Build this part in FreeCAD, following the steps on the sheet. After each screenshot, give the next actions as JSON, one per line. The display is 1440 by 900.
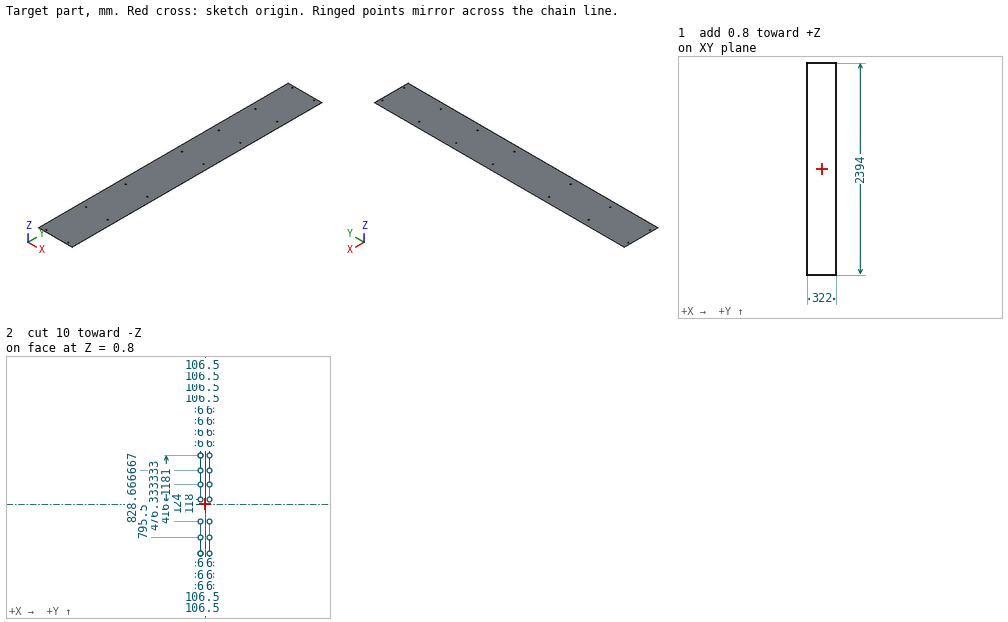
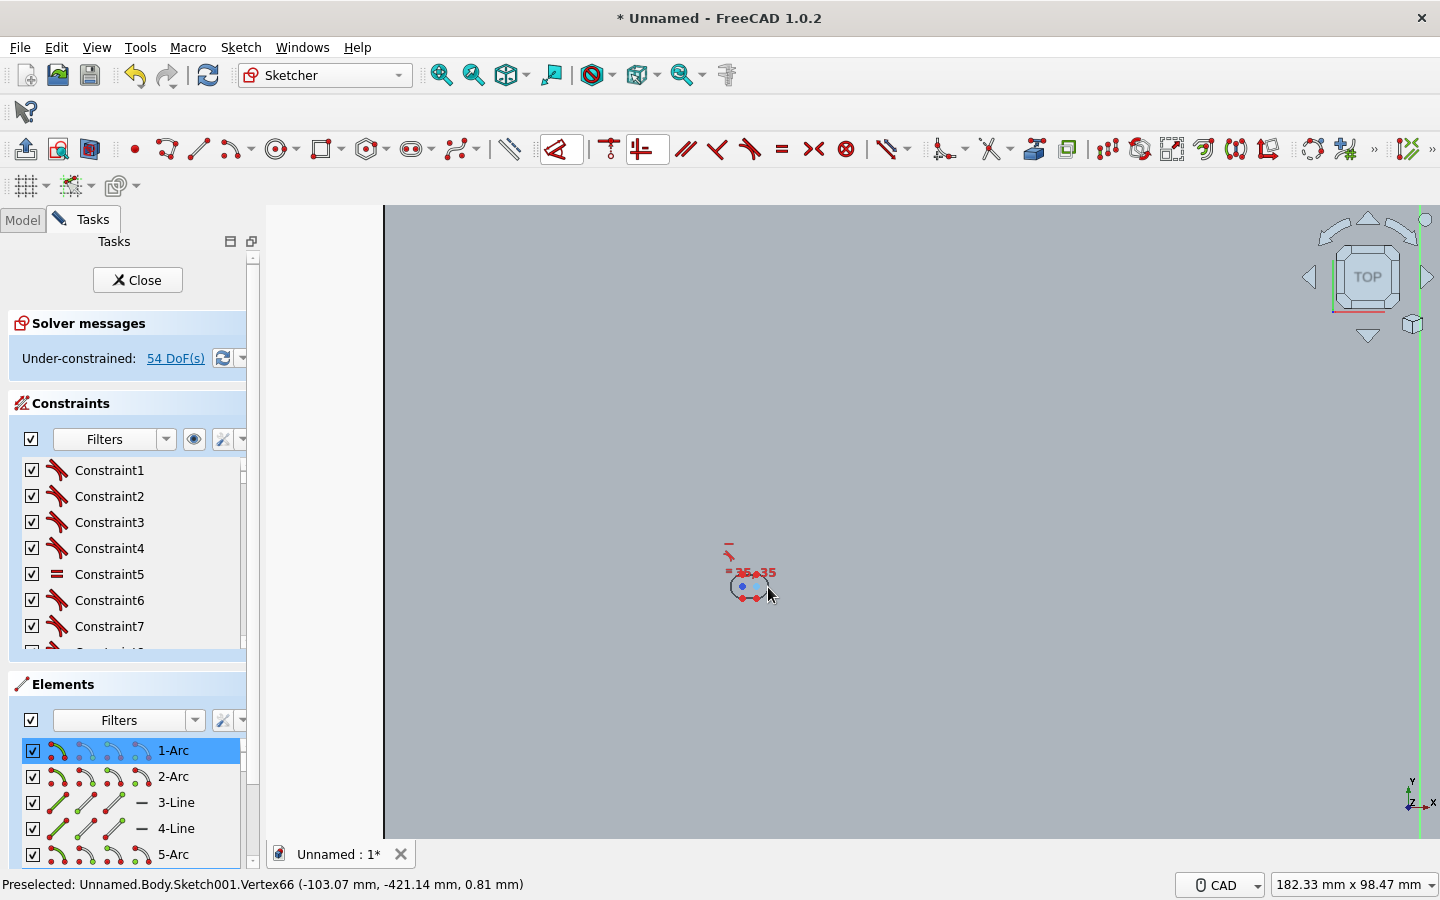
{"action": "left_click", "coordinate": [768, 586]}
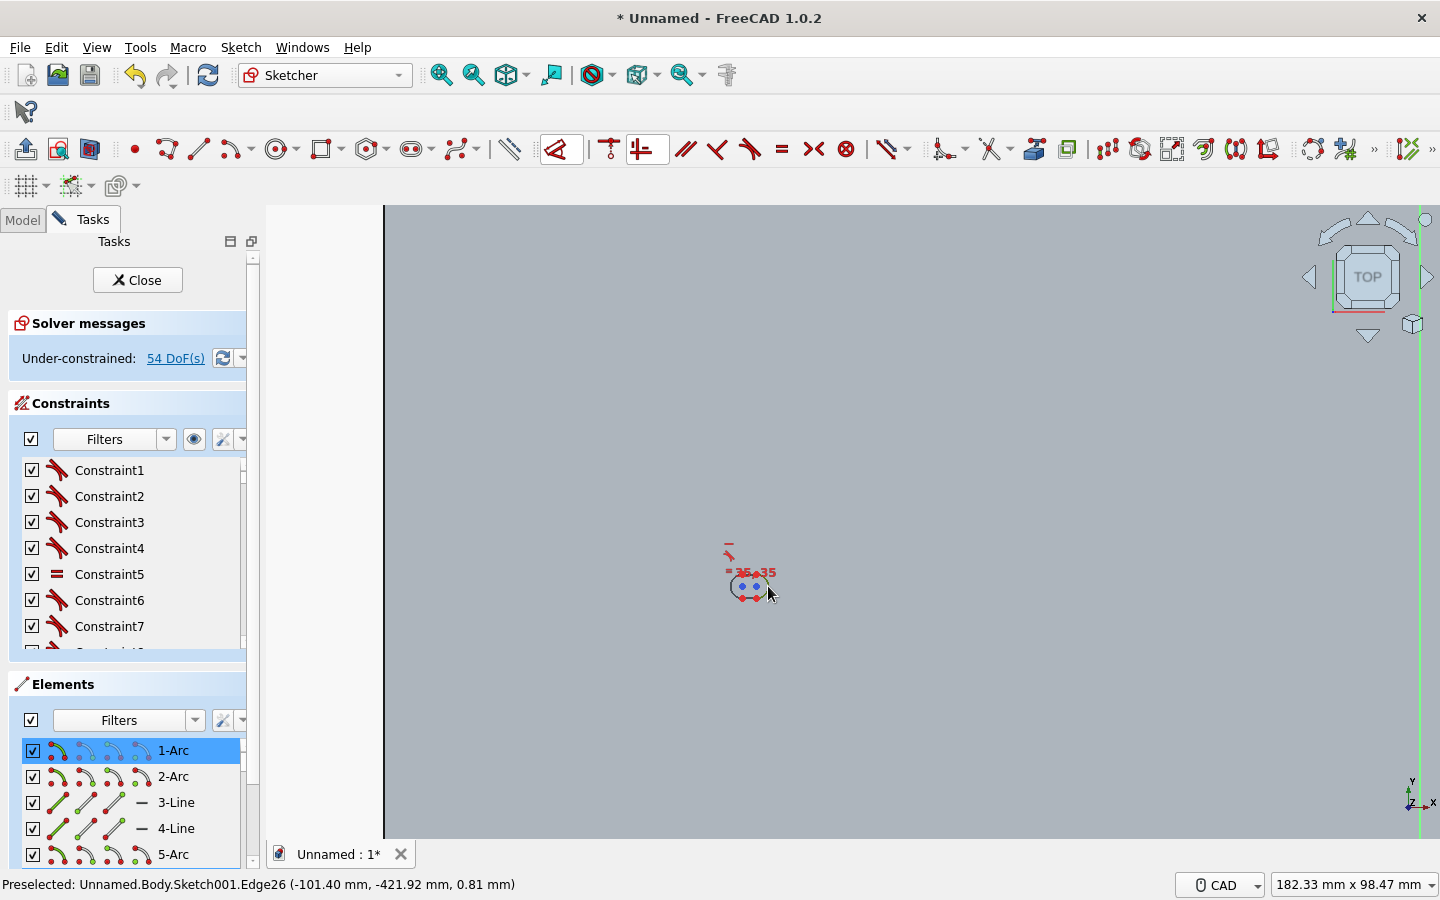
{"action": "scroll", "coordinate": [763, 613], "scroll_direction": "down", "scroll_amount": 17}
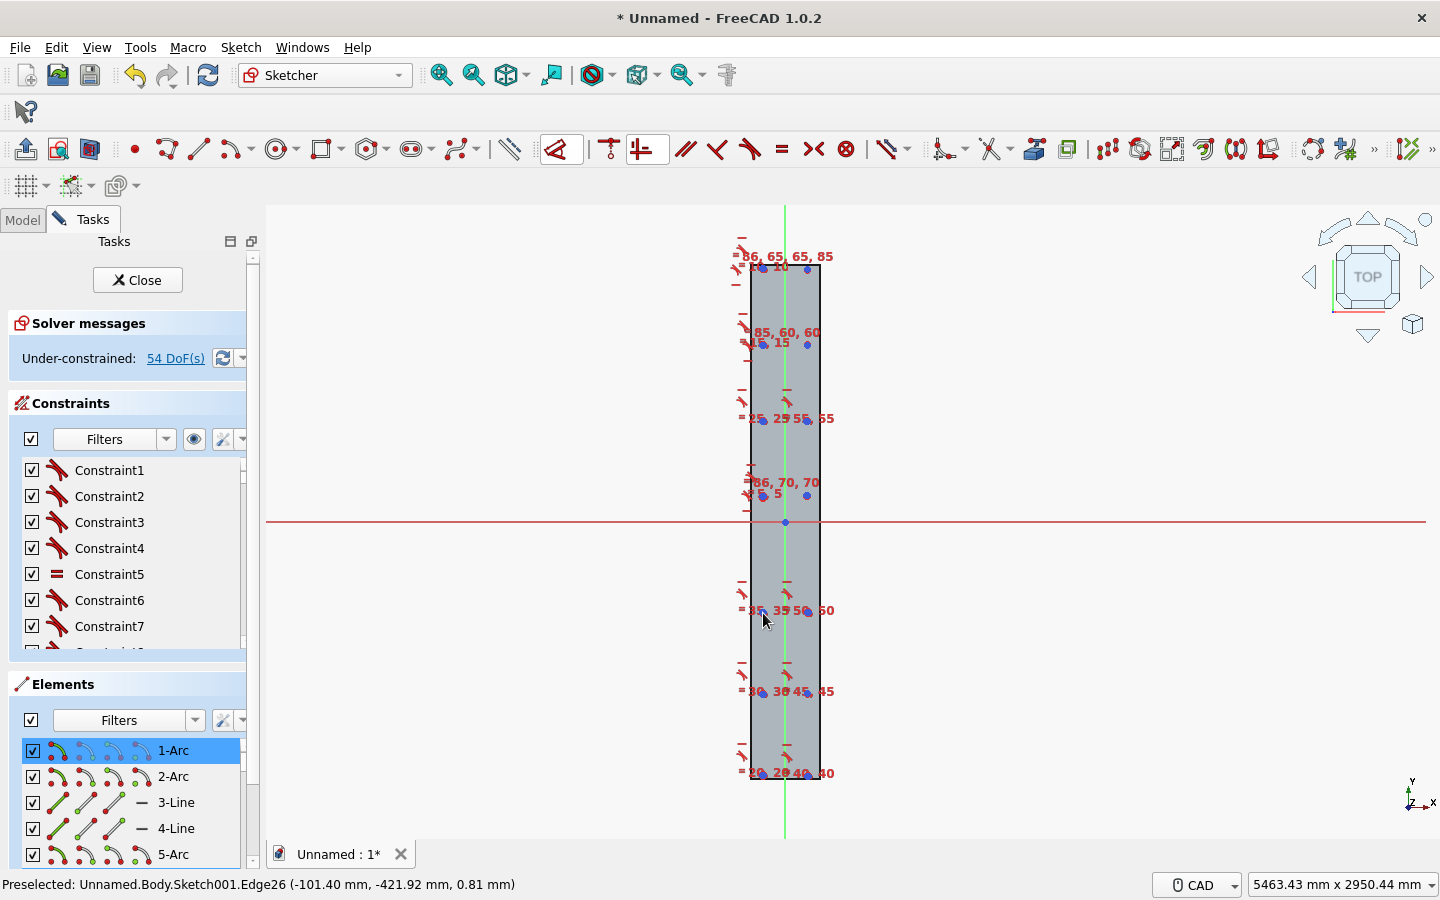
{"action": "scroll", "coordinate": [809, 777], "scroll_direction": "up", "scroll_amount": 13}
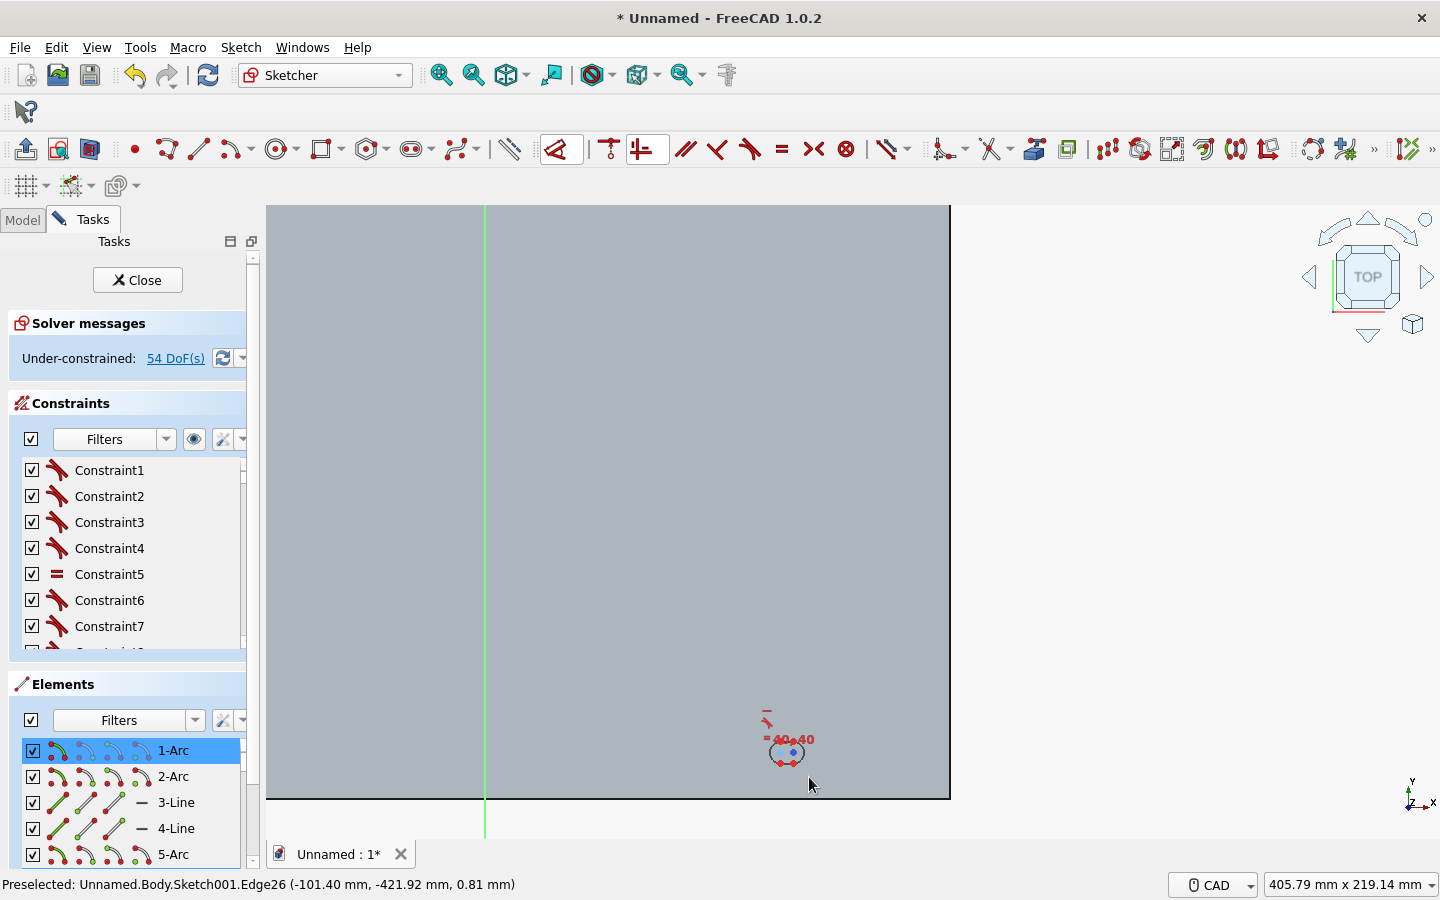
{"action": "left_click", "coordinate": [802, 759]}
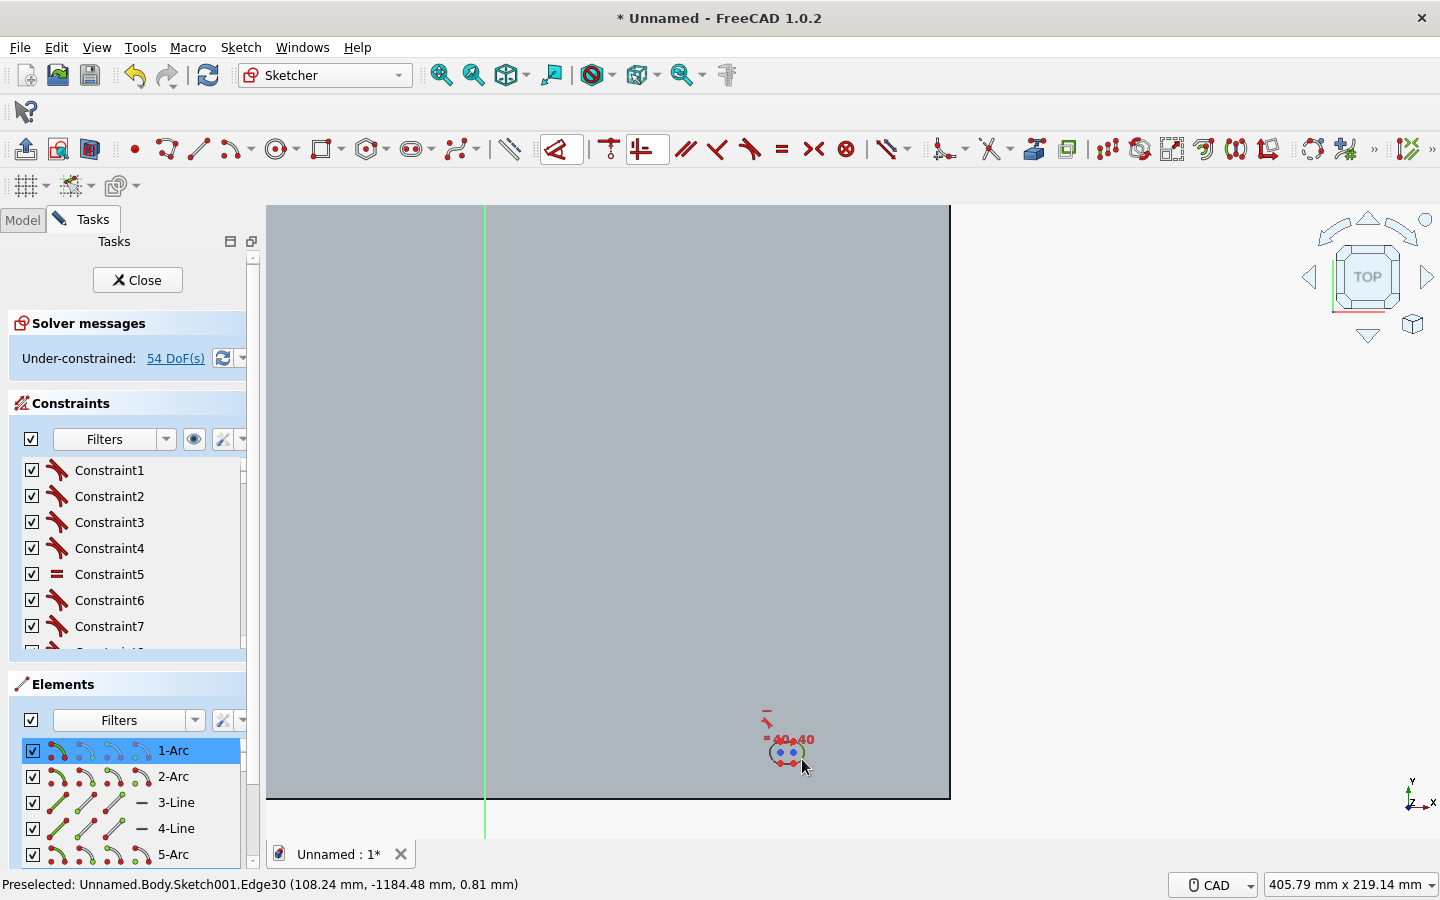
{"action": "scroll", "coordinate": [804, 728], "scroll_direction": "down", "scroll_amount": 14}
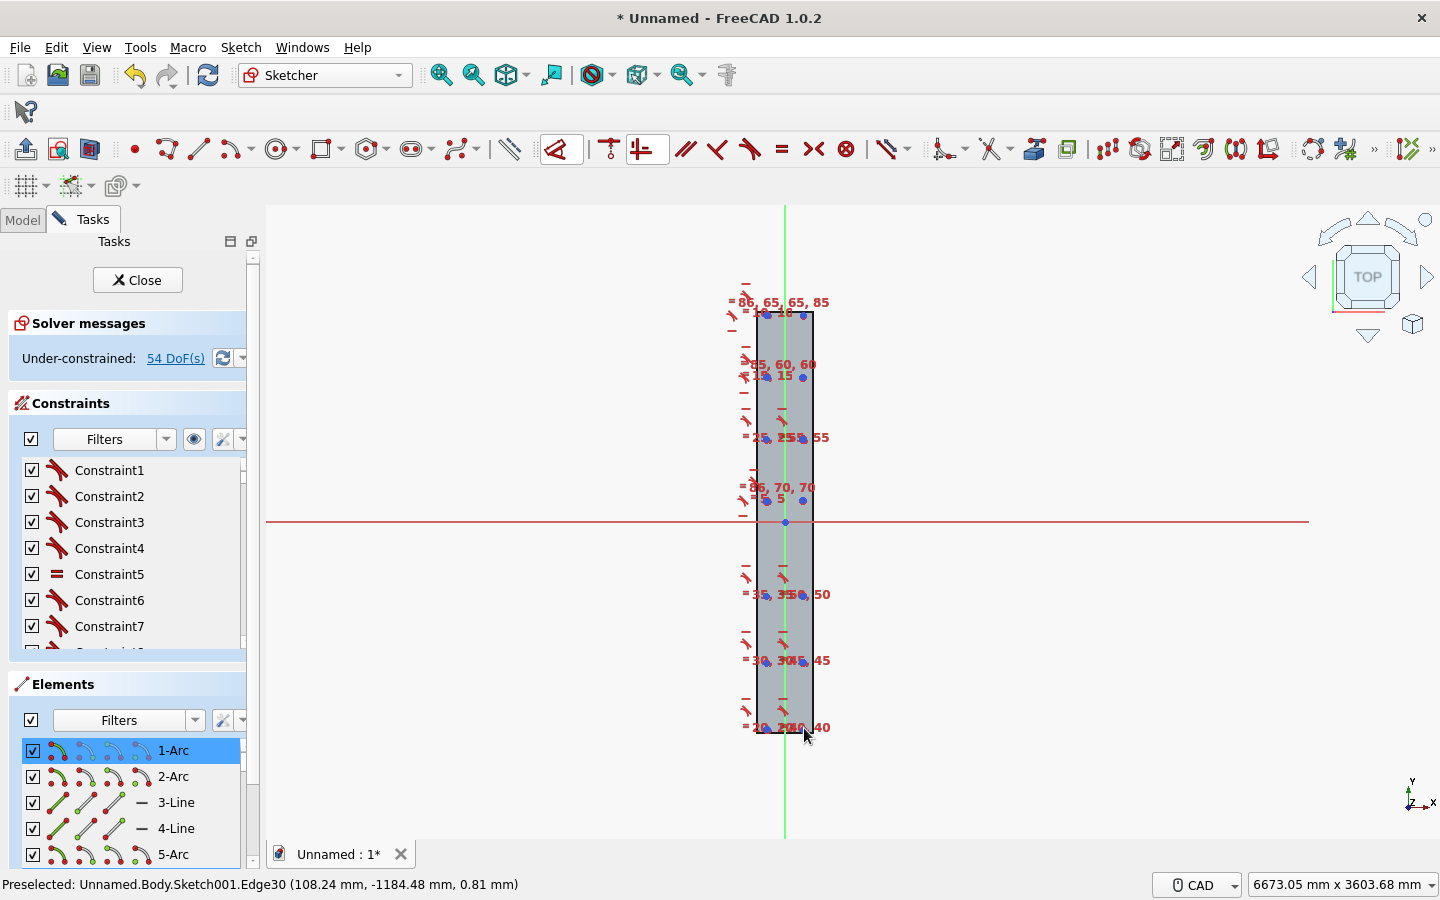
{"action": "scroll", "coordinate": [804, 663], "scroll_direction": "up", "scroll_amount": 14}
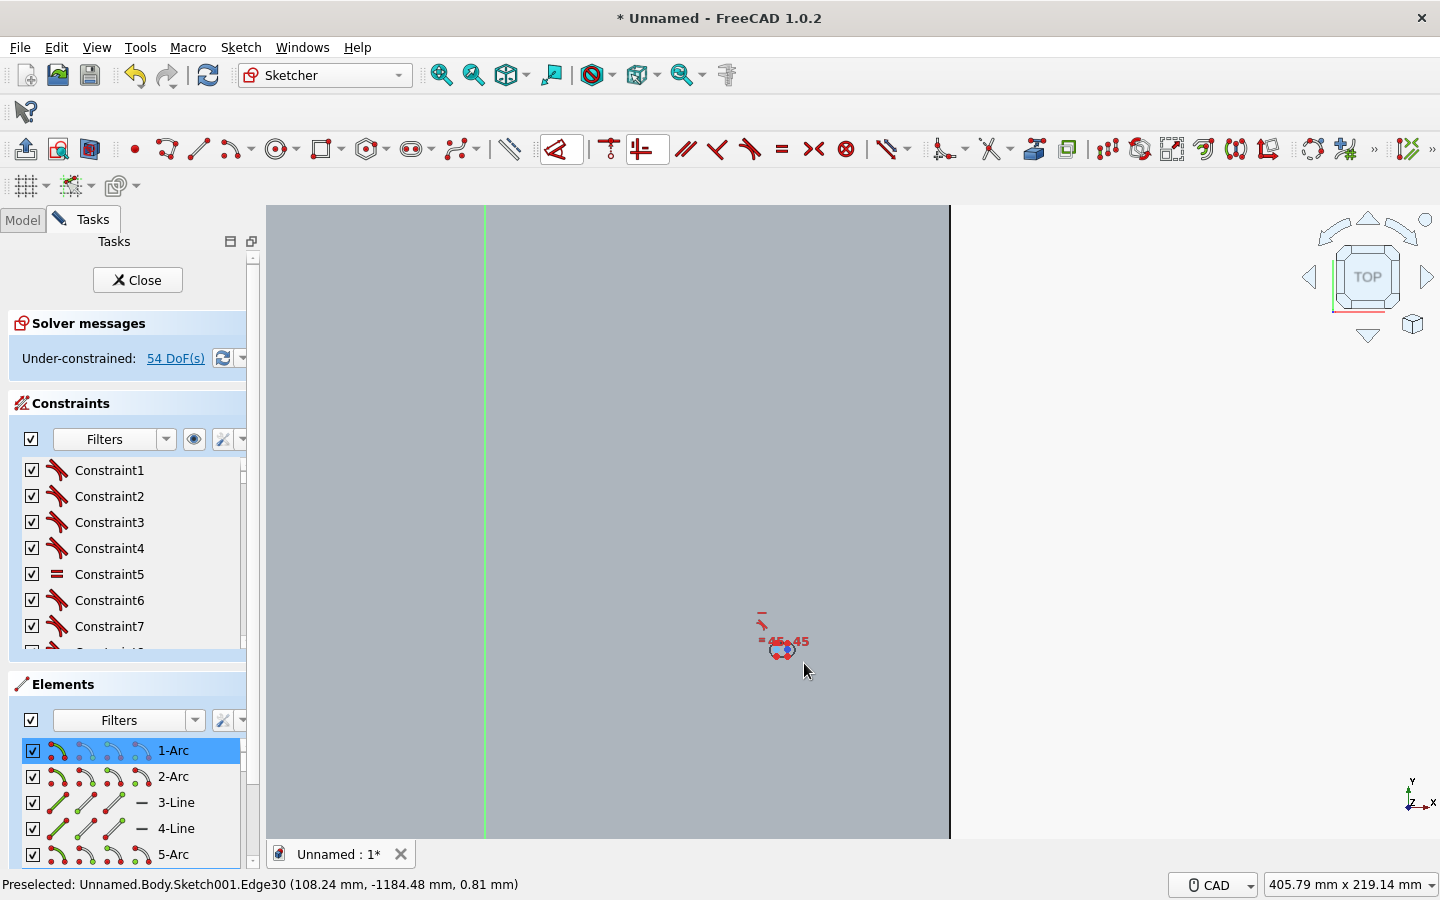
{"action": "left_click", "coordinate": [795, 650]}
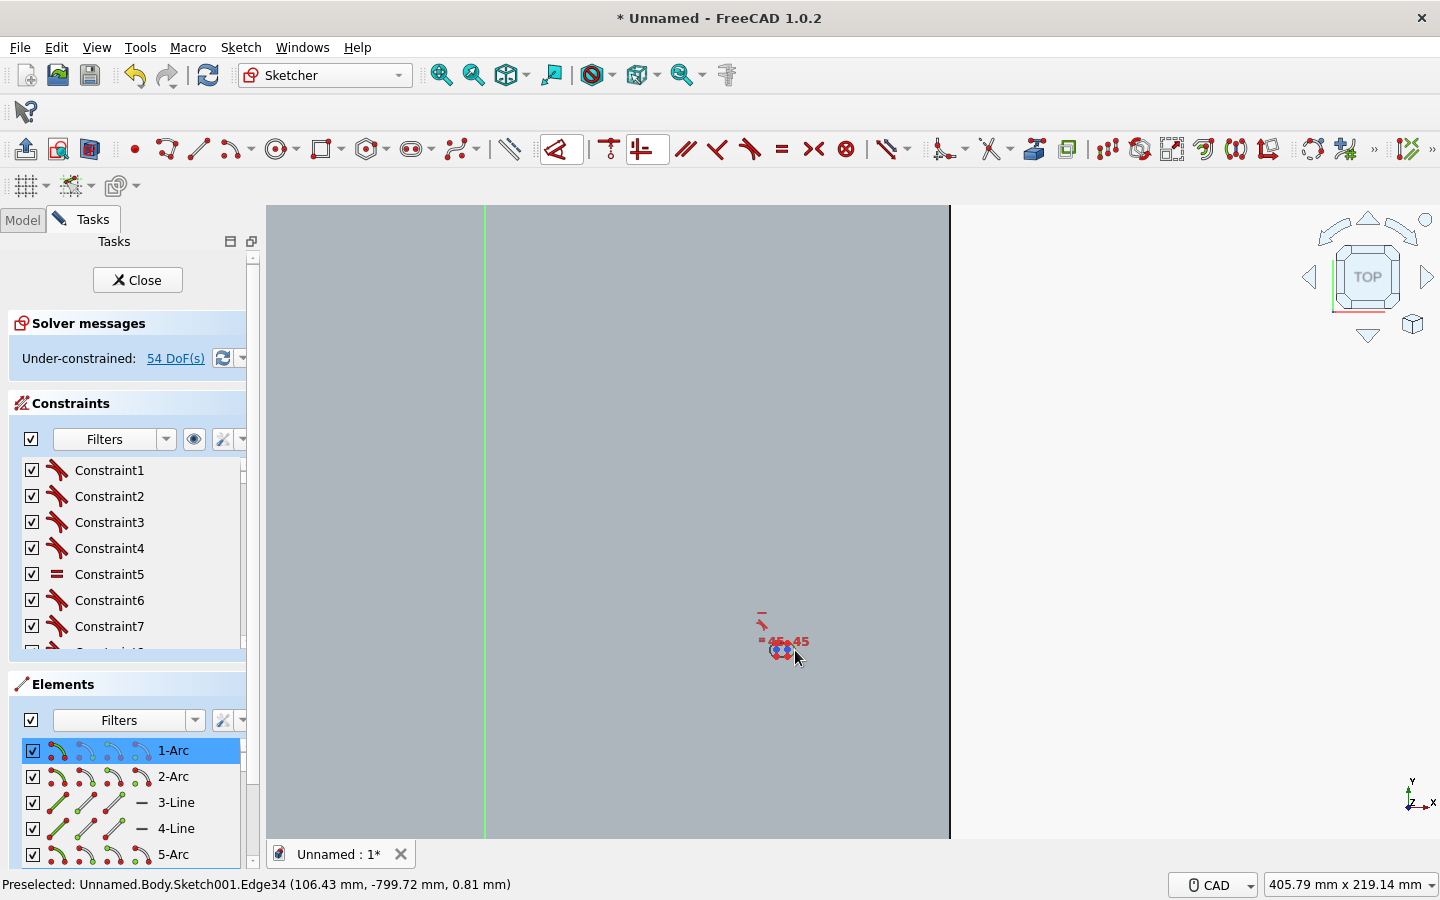
{"action": "scroll", "coordinate": [804, 663], "scroll_direction": "down", "scroll_amount": 14}